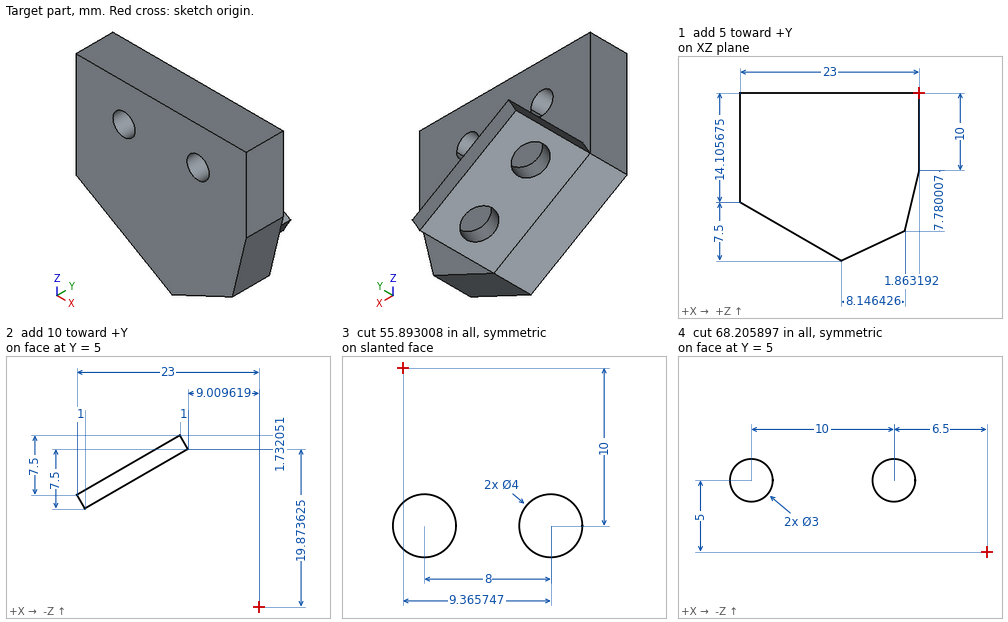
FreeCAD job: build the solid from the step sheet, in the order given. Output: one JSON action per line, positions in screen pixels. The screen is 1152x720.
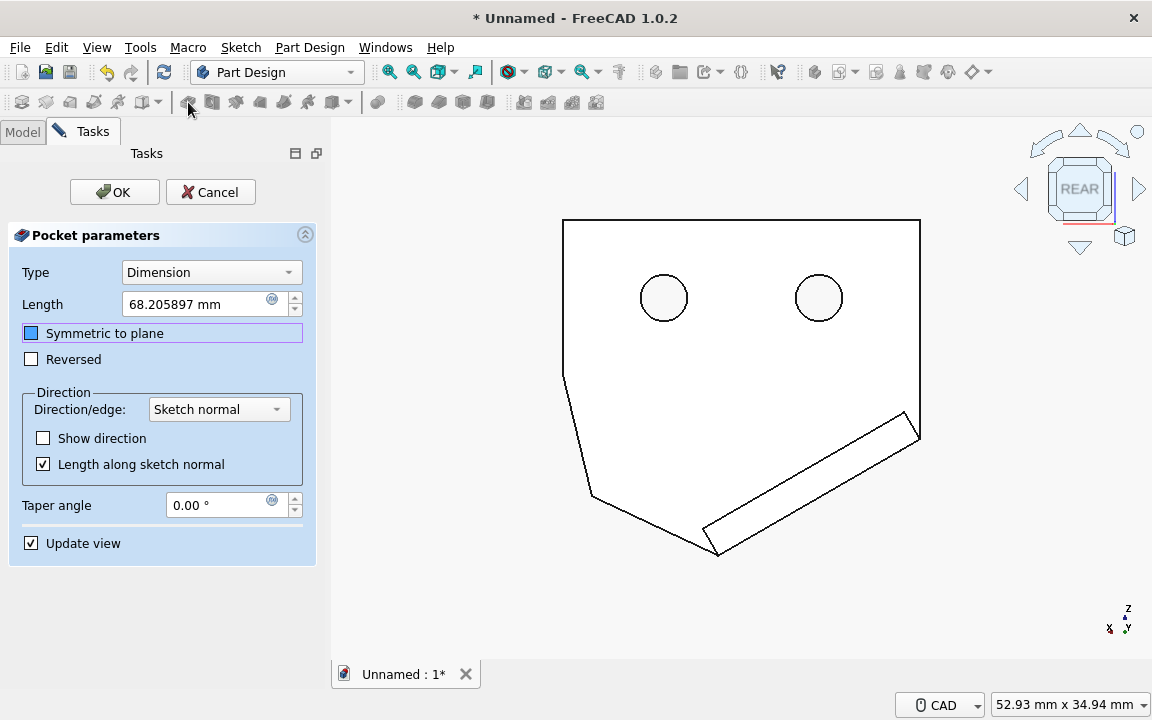
{"action": "left_click", "coordinate": [30, 333]}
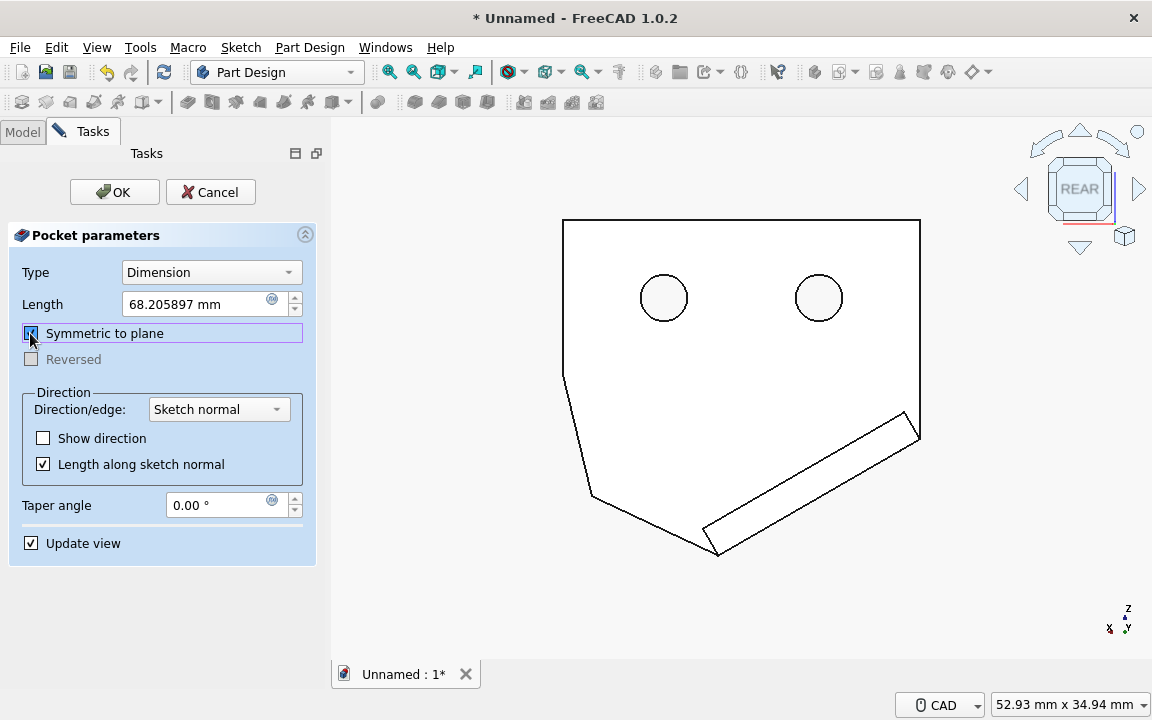
{"action": "left_click", "coordinate": [115, 192]}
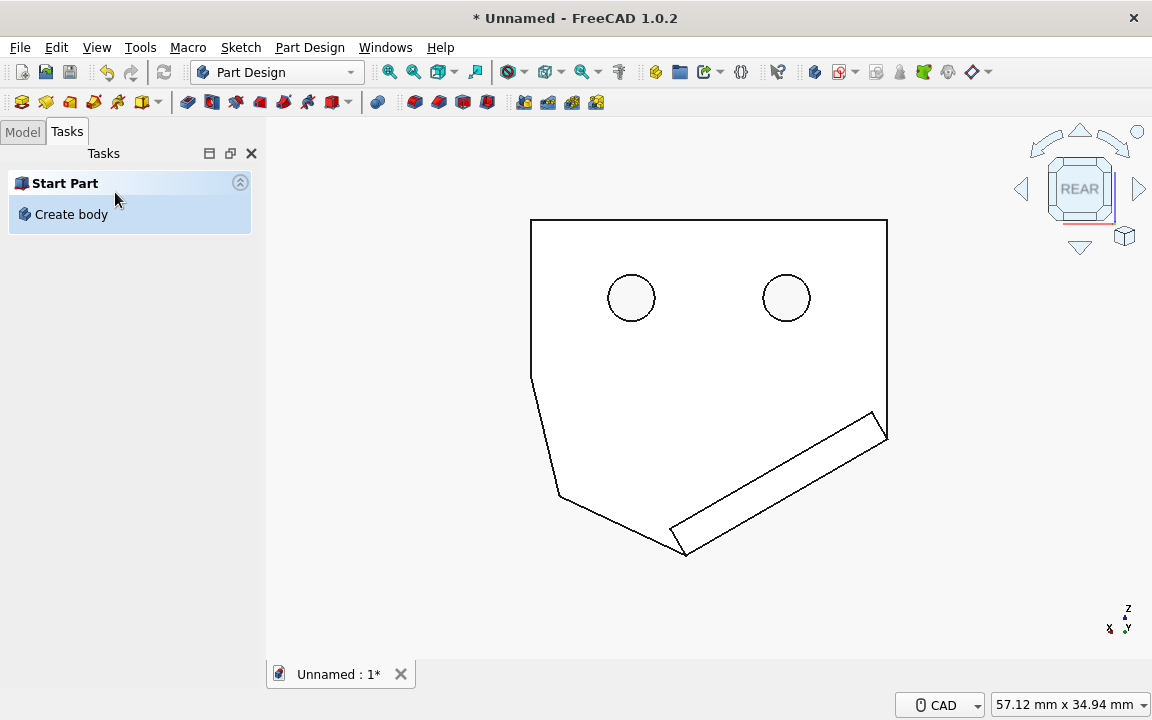
{"action": "key", "text": "0"}